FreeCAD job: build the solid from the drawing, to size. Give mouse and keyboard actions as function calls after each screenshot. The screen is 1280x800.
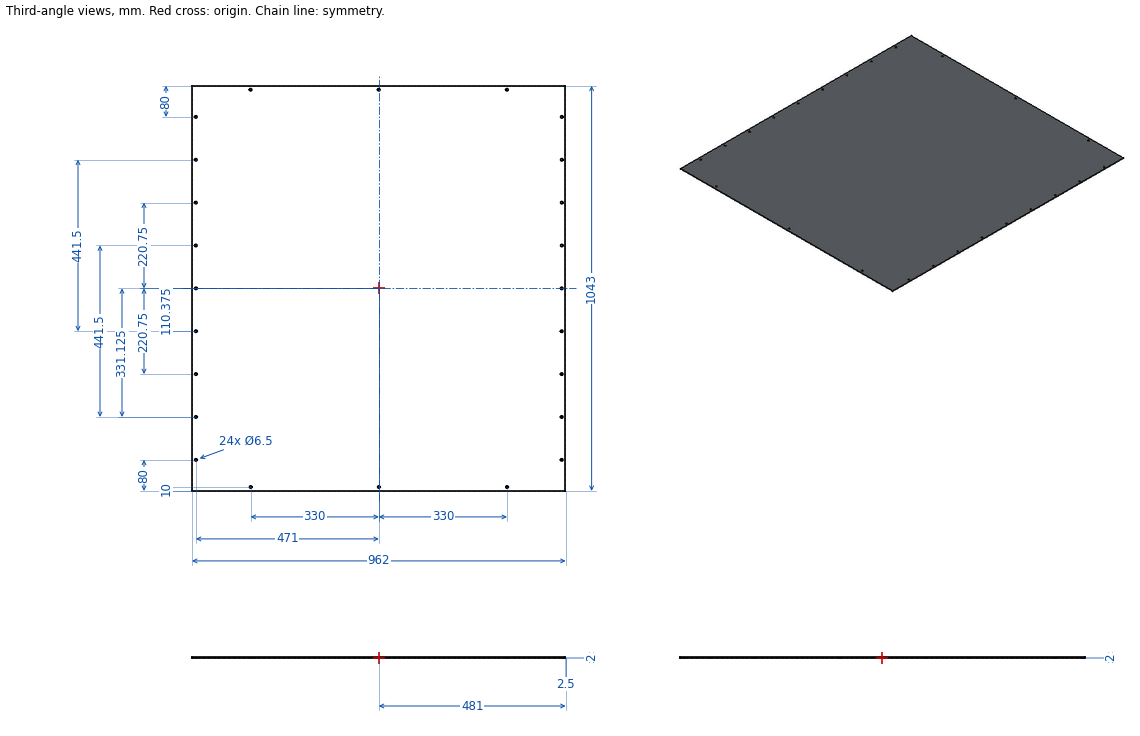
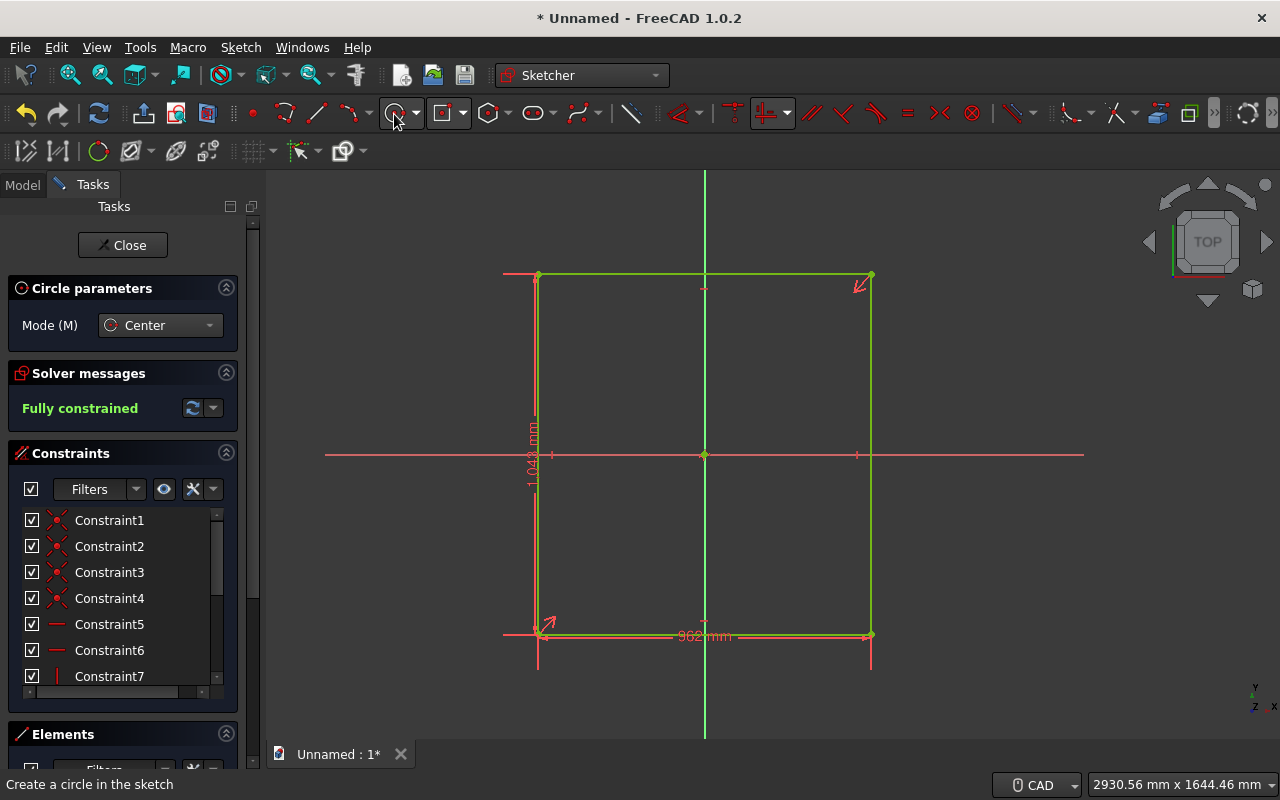
scroll(542, 607, up, 16)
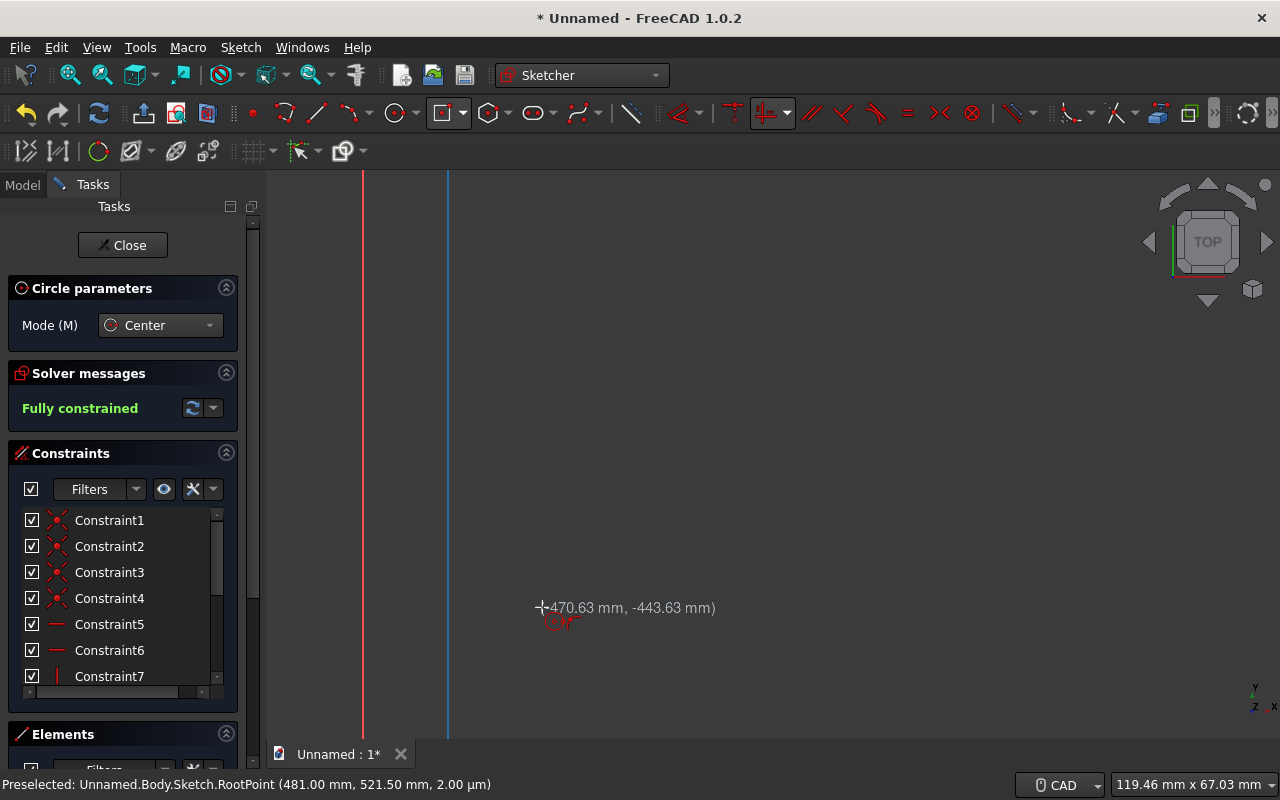
scroll(504, 643, down, 15)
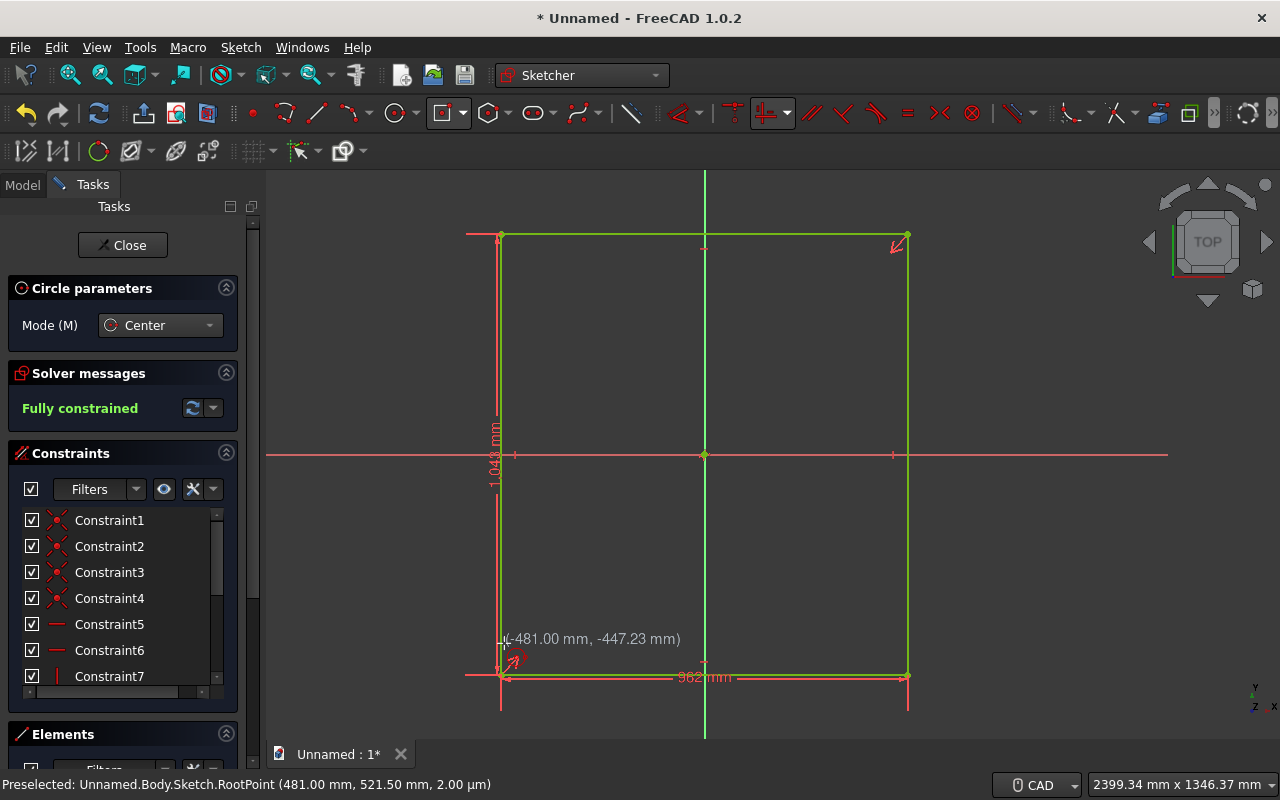
scroll(506, 641, up, 7)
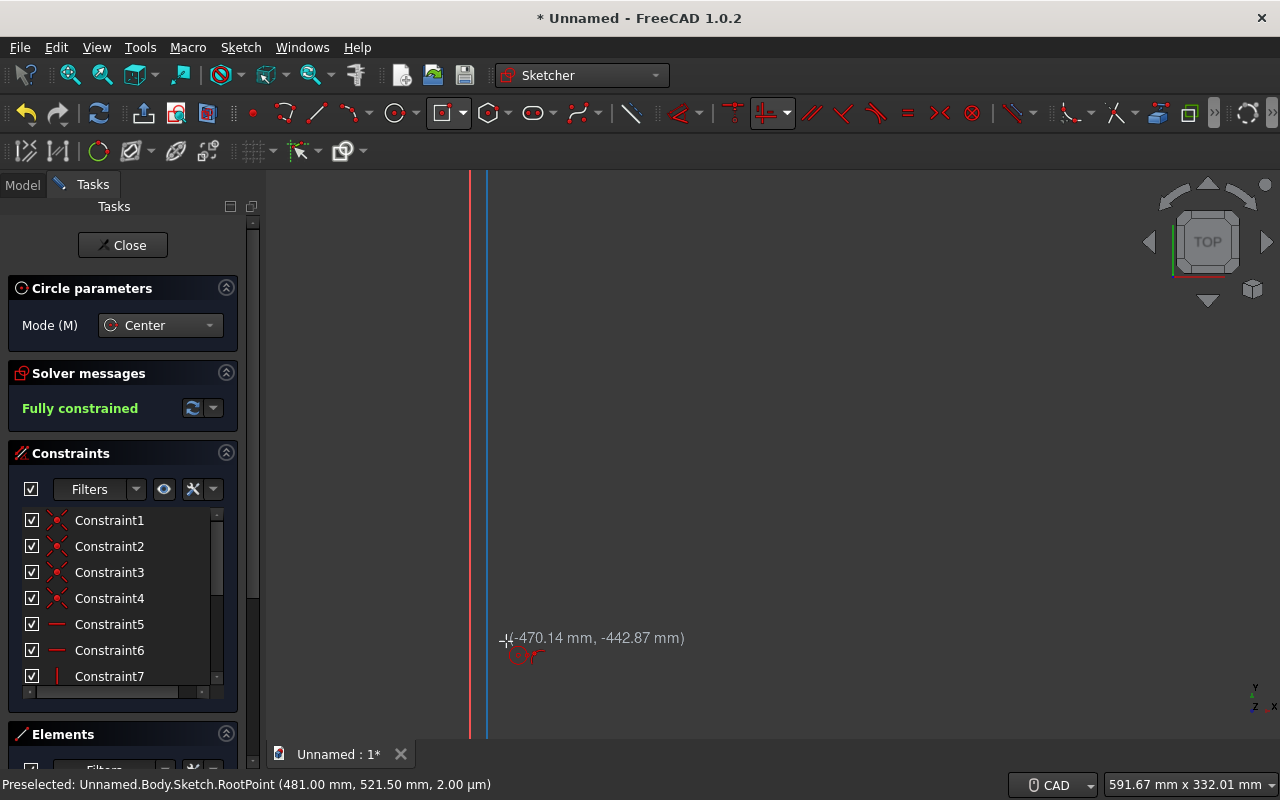
click(504, 640)
move(508, 636)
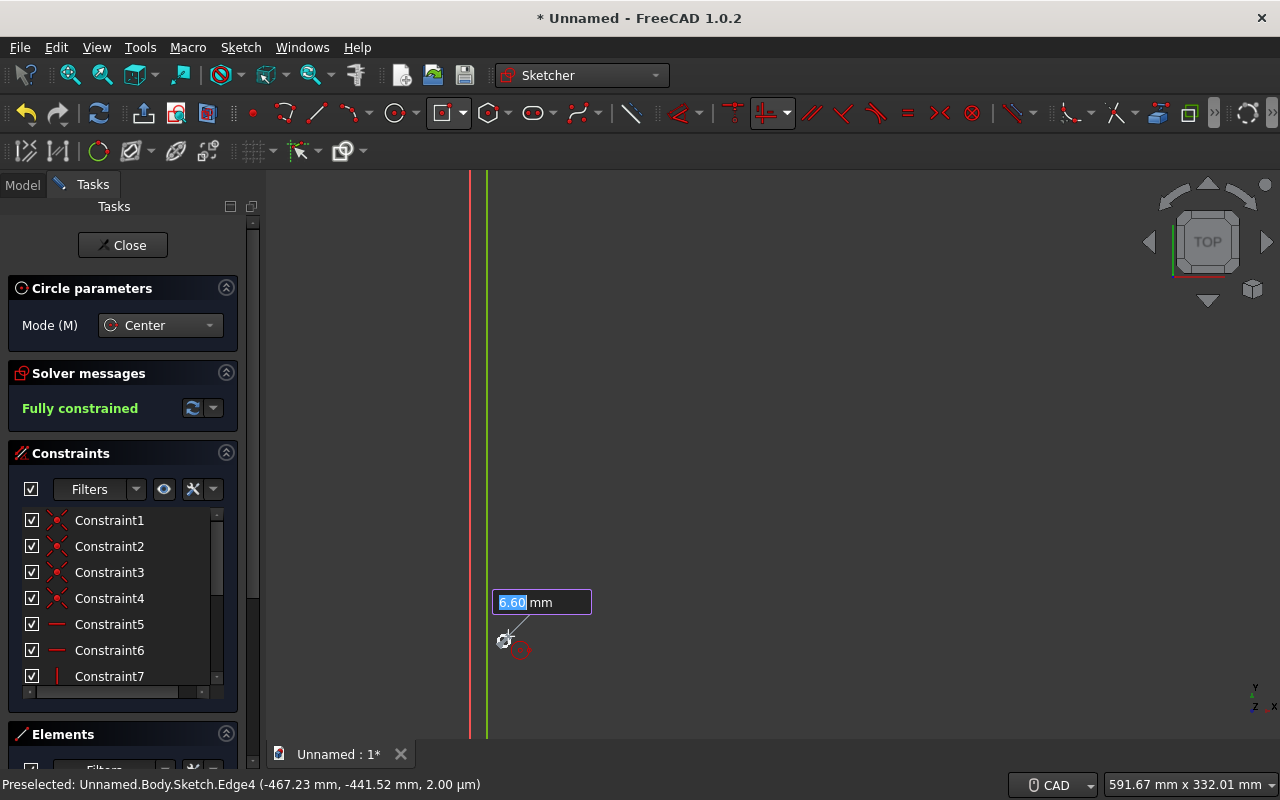
text(6.5)
key(Return)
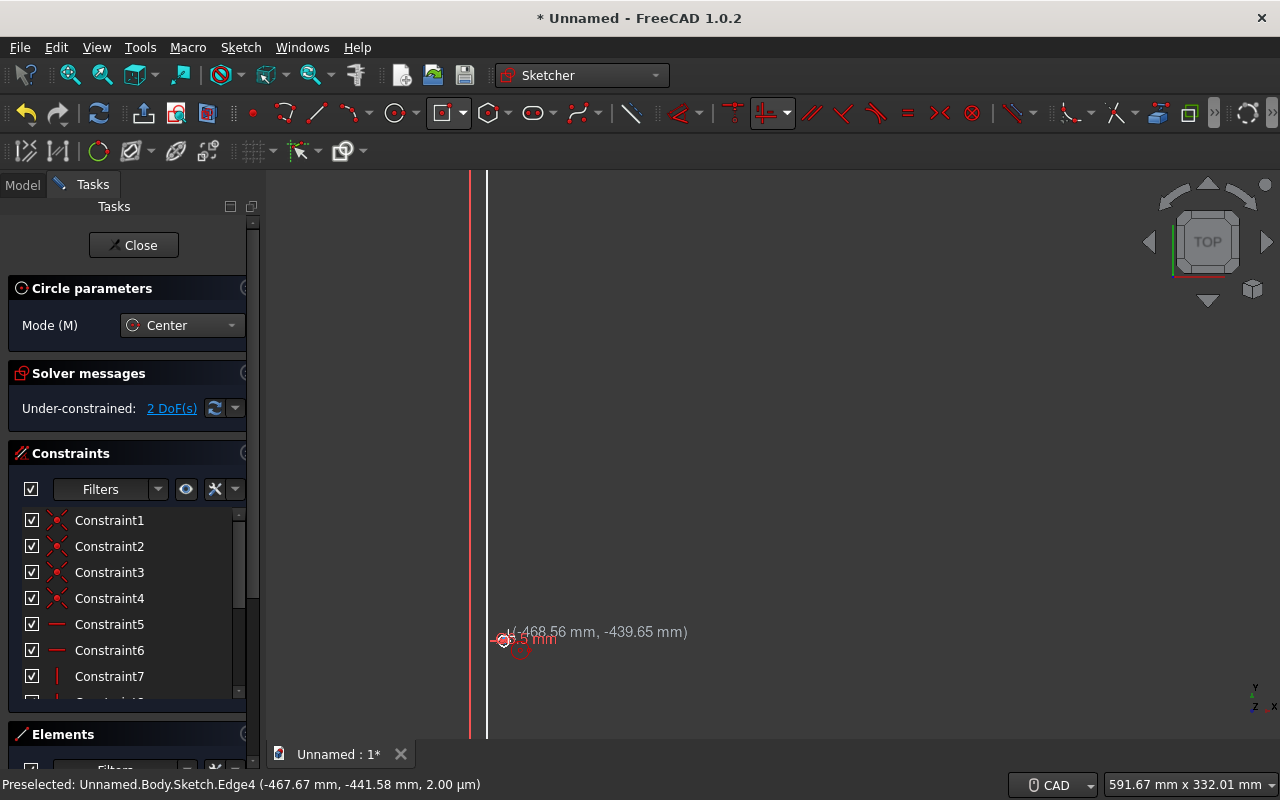
scroll(551, 599, down, 8)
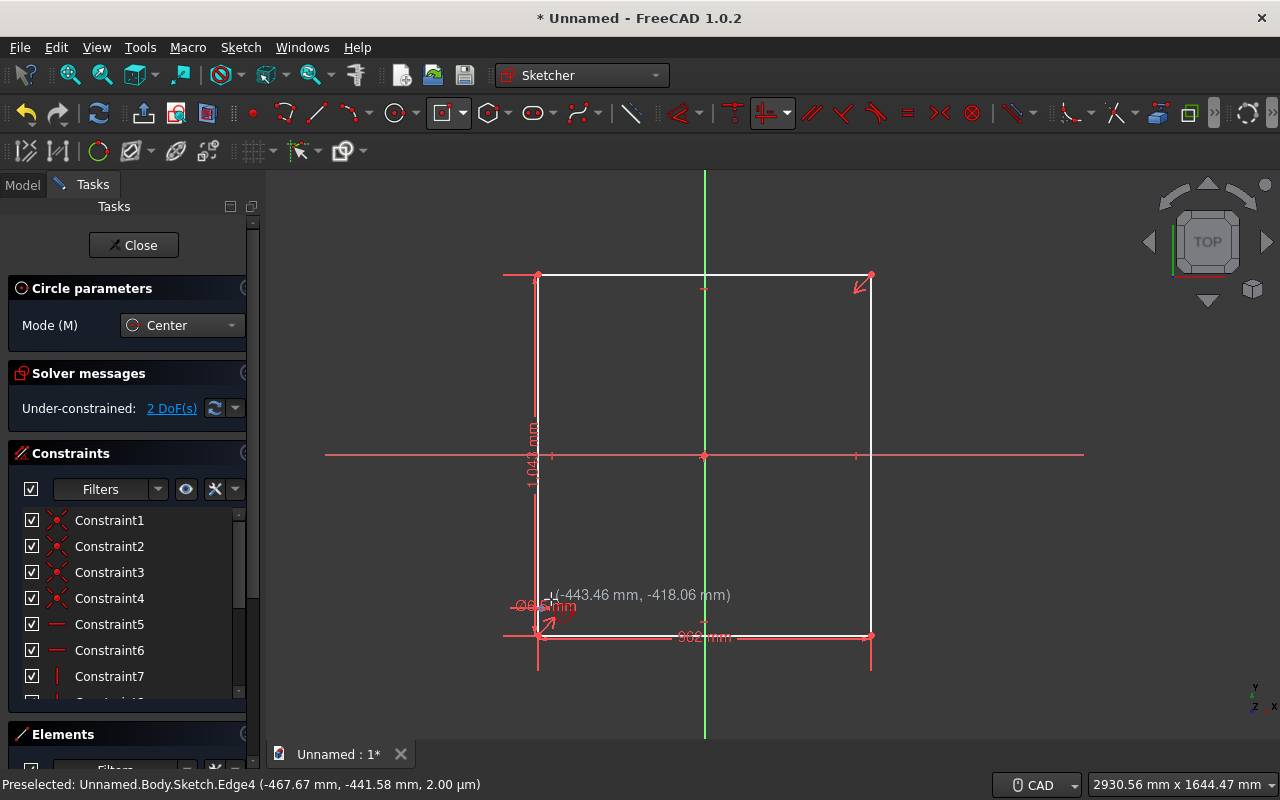
scroll(590, 632, up, 16)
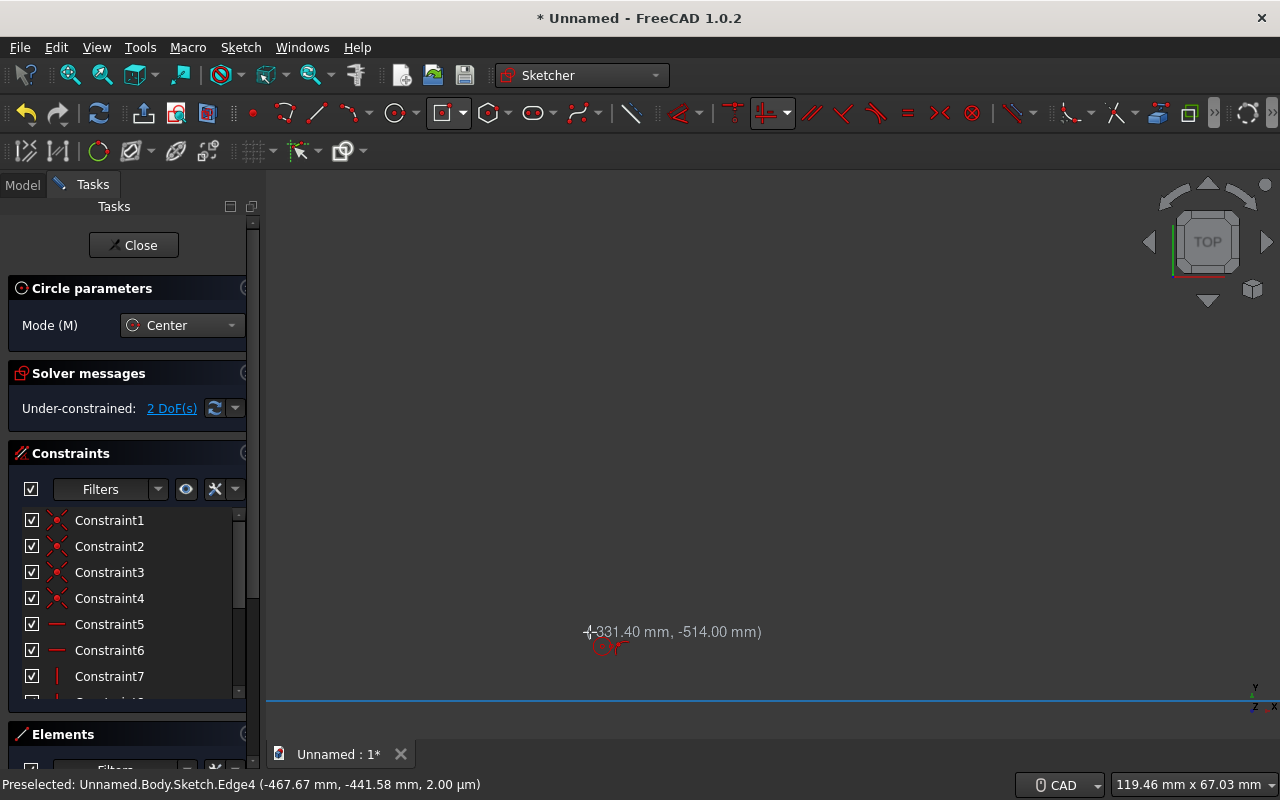
scroll(564, 674, down, 15)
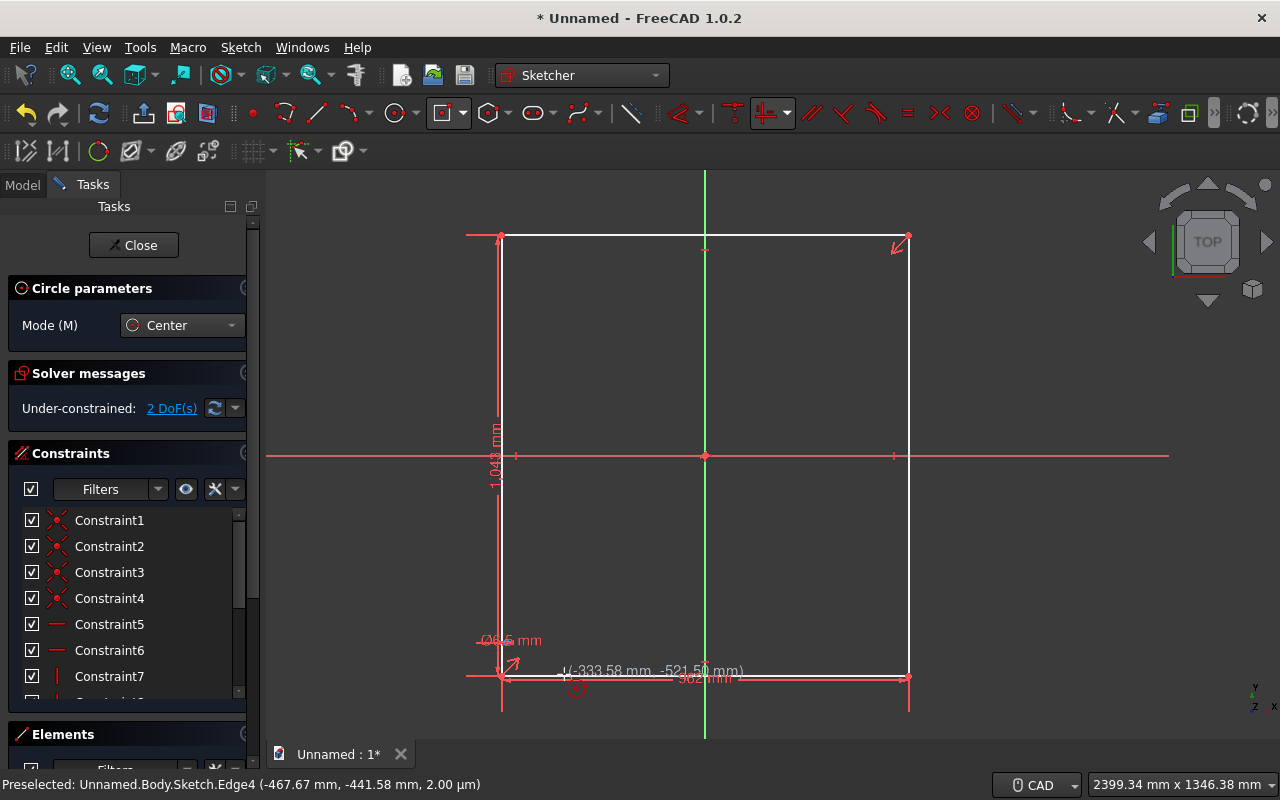
scroll(566, 672, up, 7)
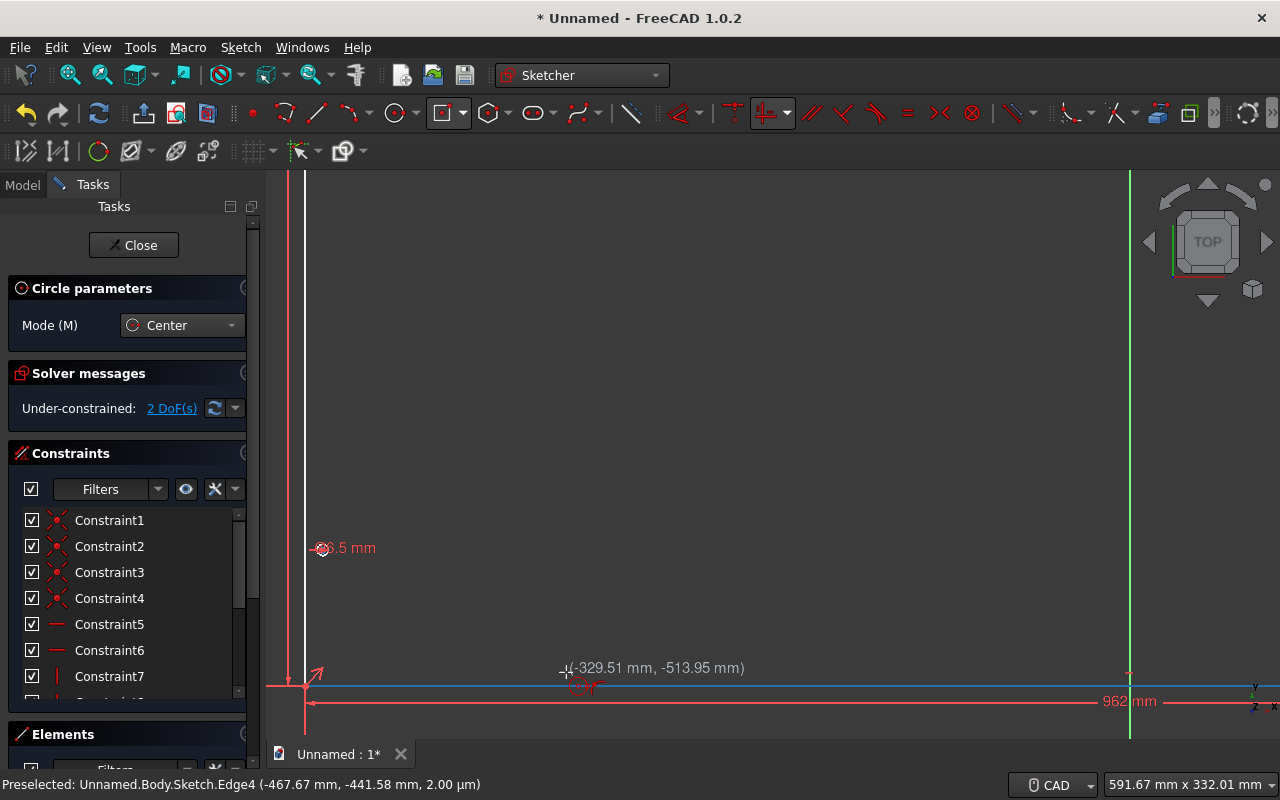
click(564, 669)
move(568, 665)